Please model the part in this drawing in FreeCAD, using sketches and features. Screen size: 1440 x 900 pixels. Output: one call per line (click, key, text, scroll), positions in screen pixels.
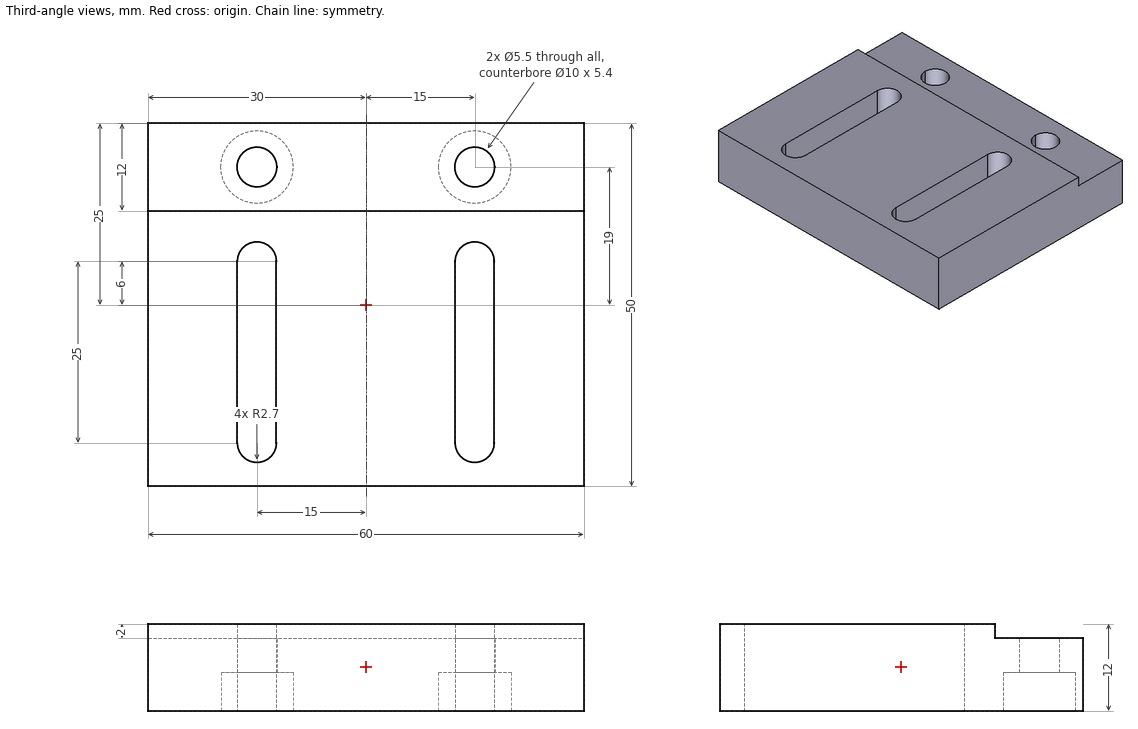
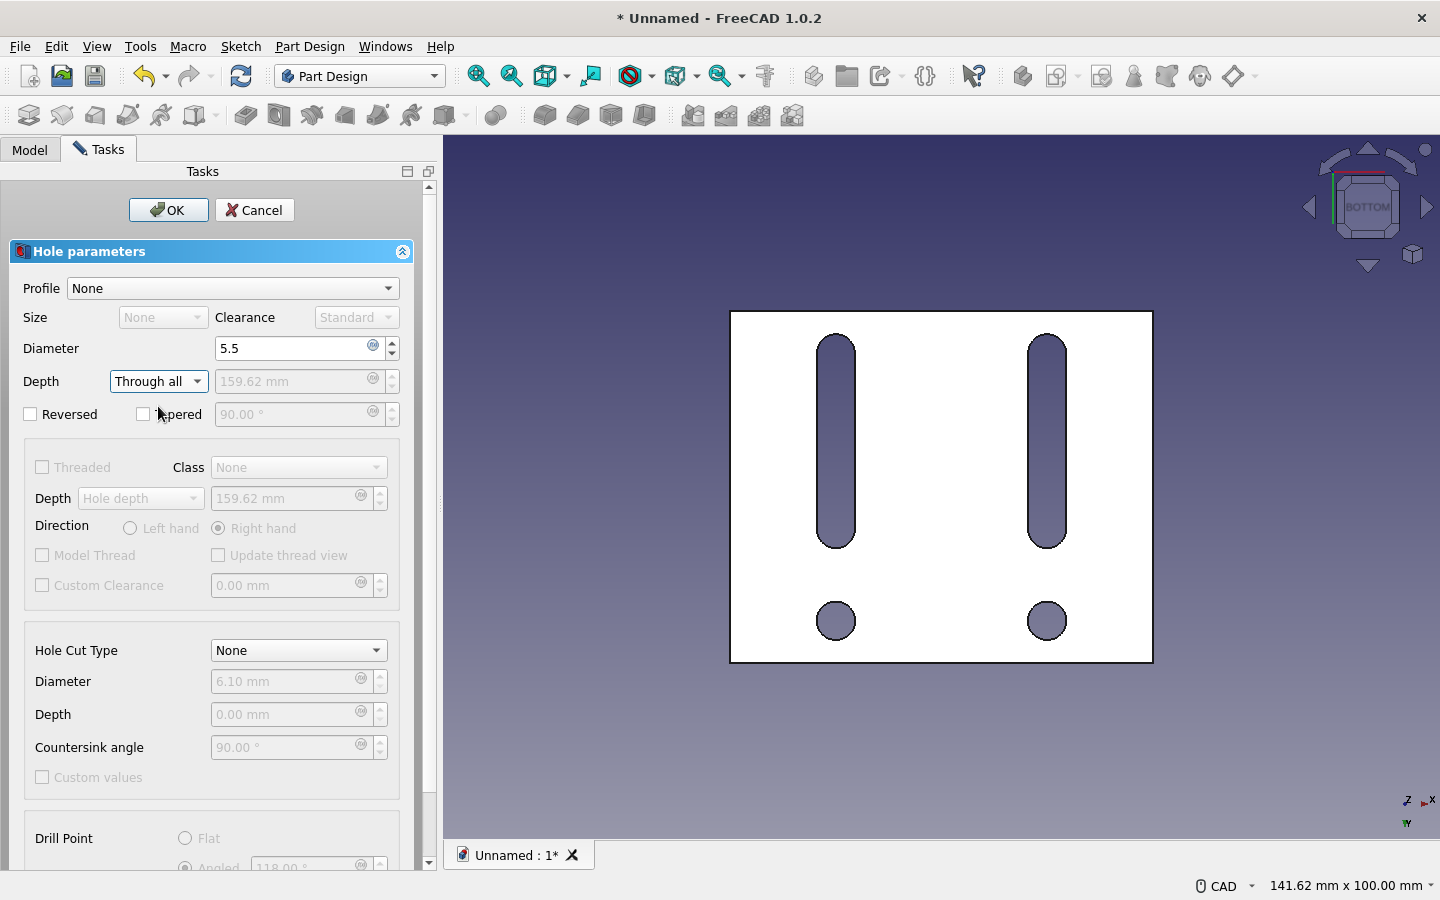
click(300, 650)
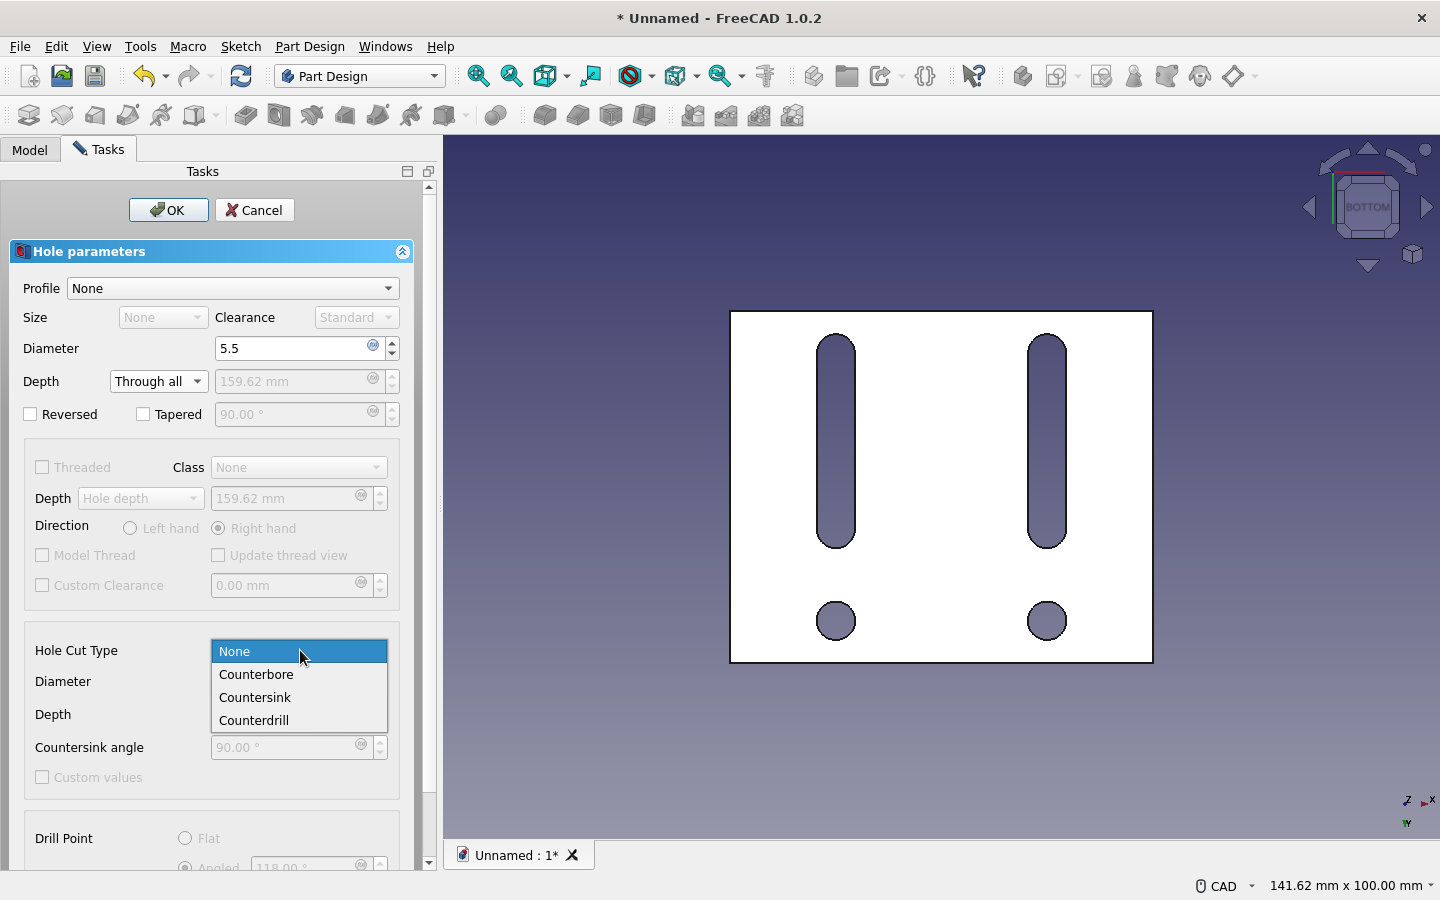
click(298, 674)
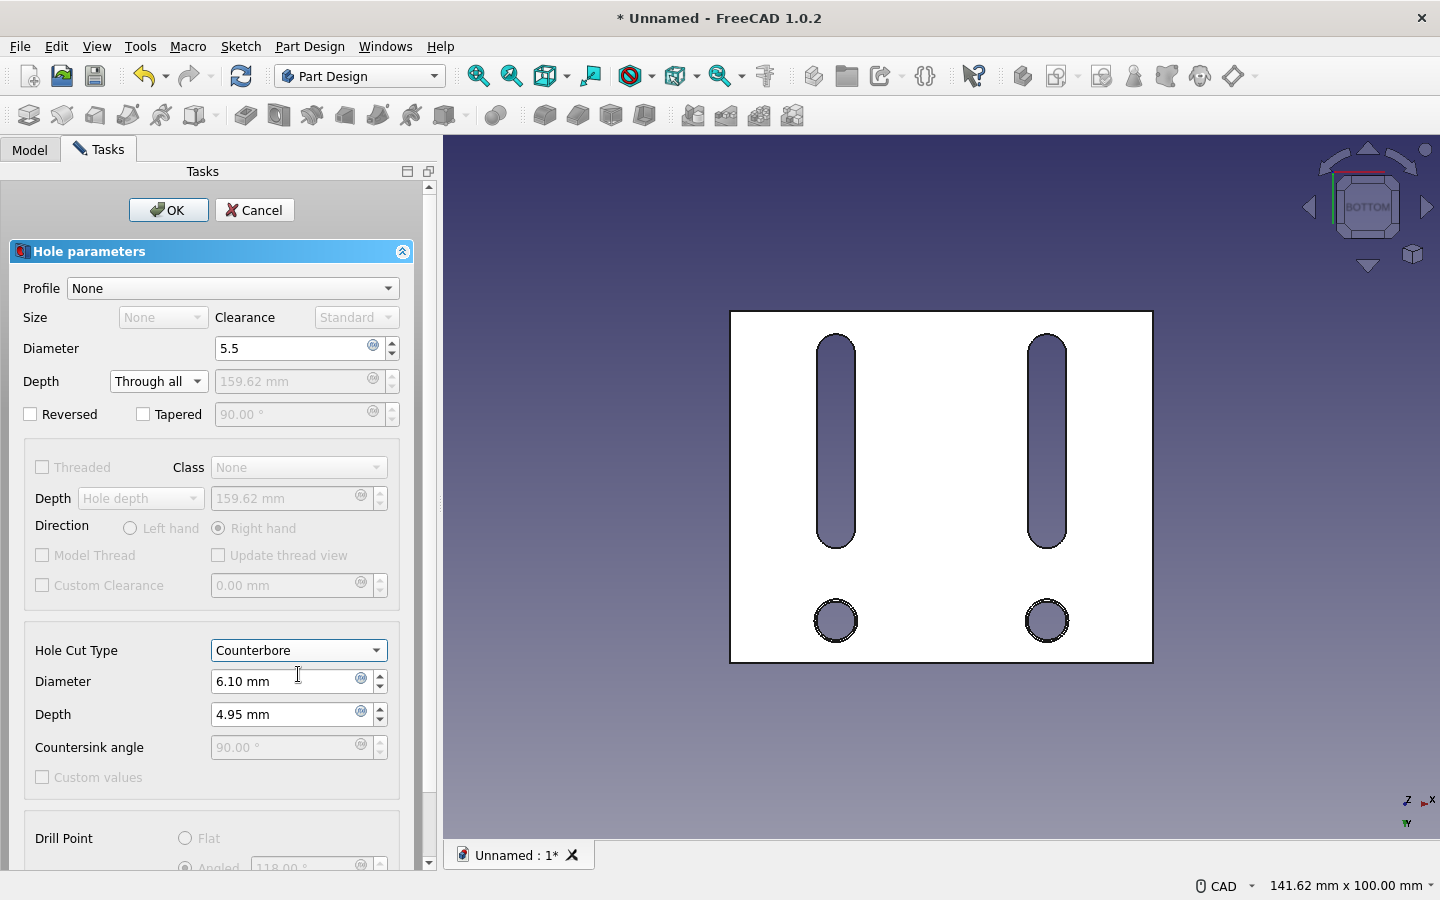
triple_click(292, 682)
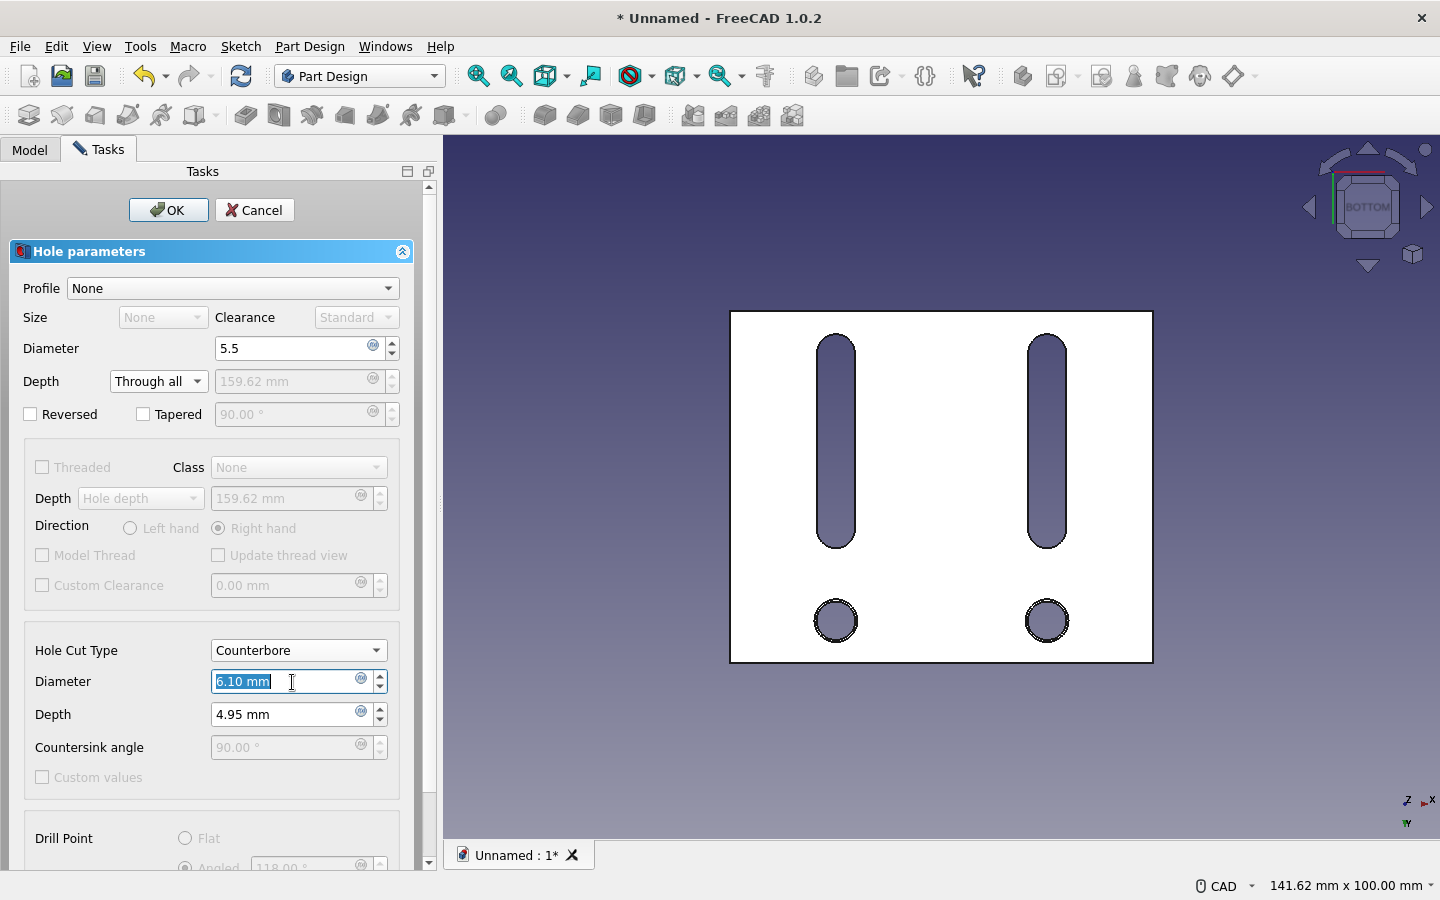
text(10)
key(Tab)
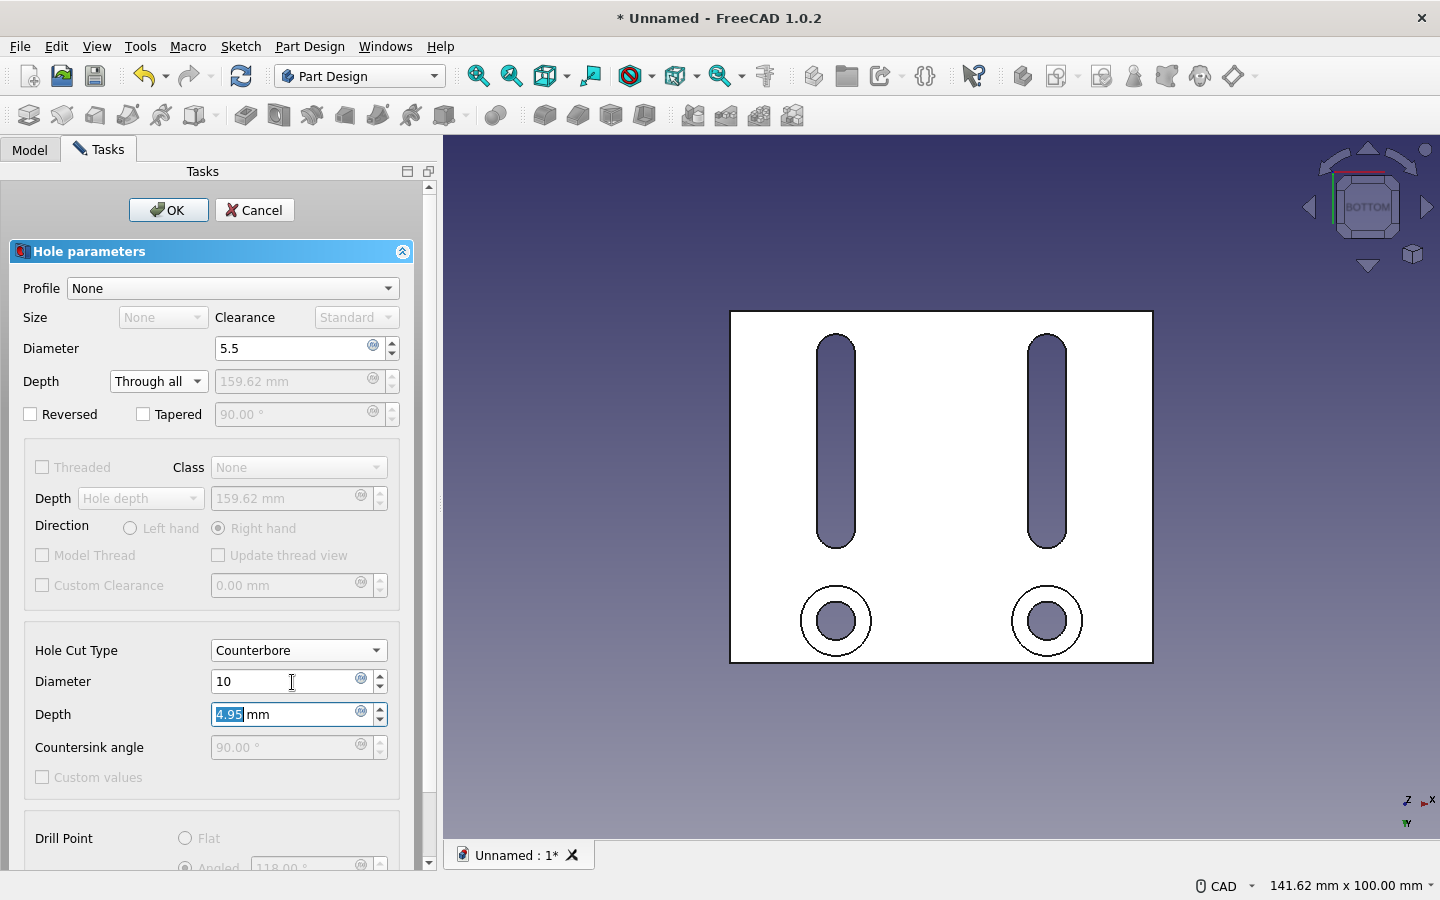
text(5.4)
key(Tab)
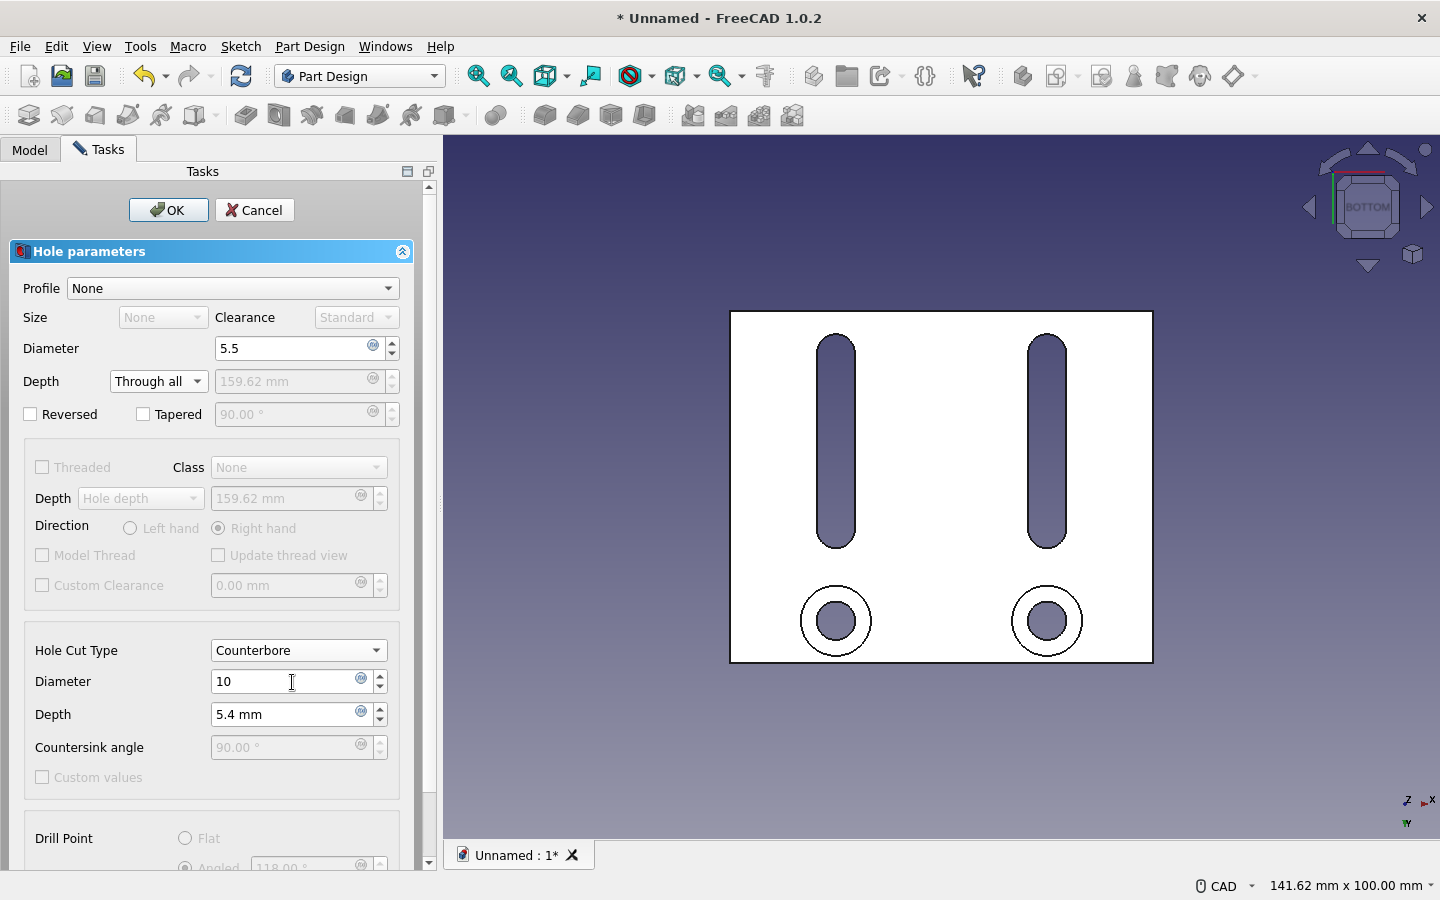
click(169, 210)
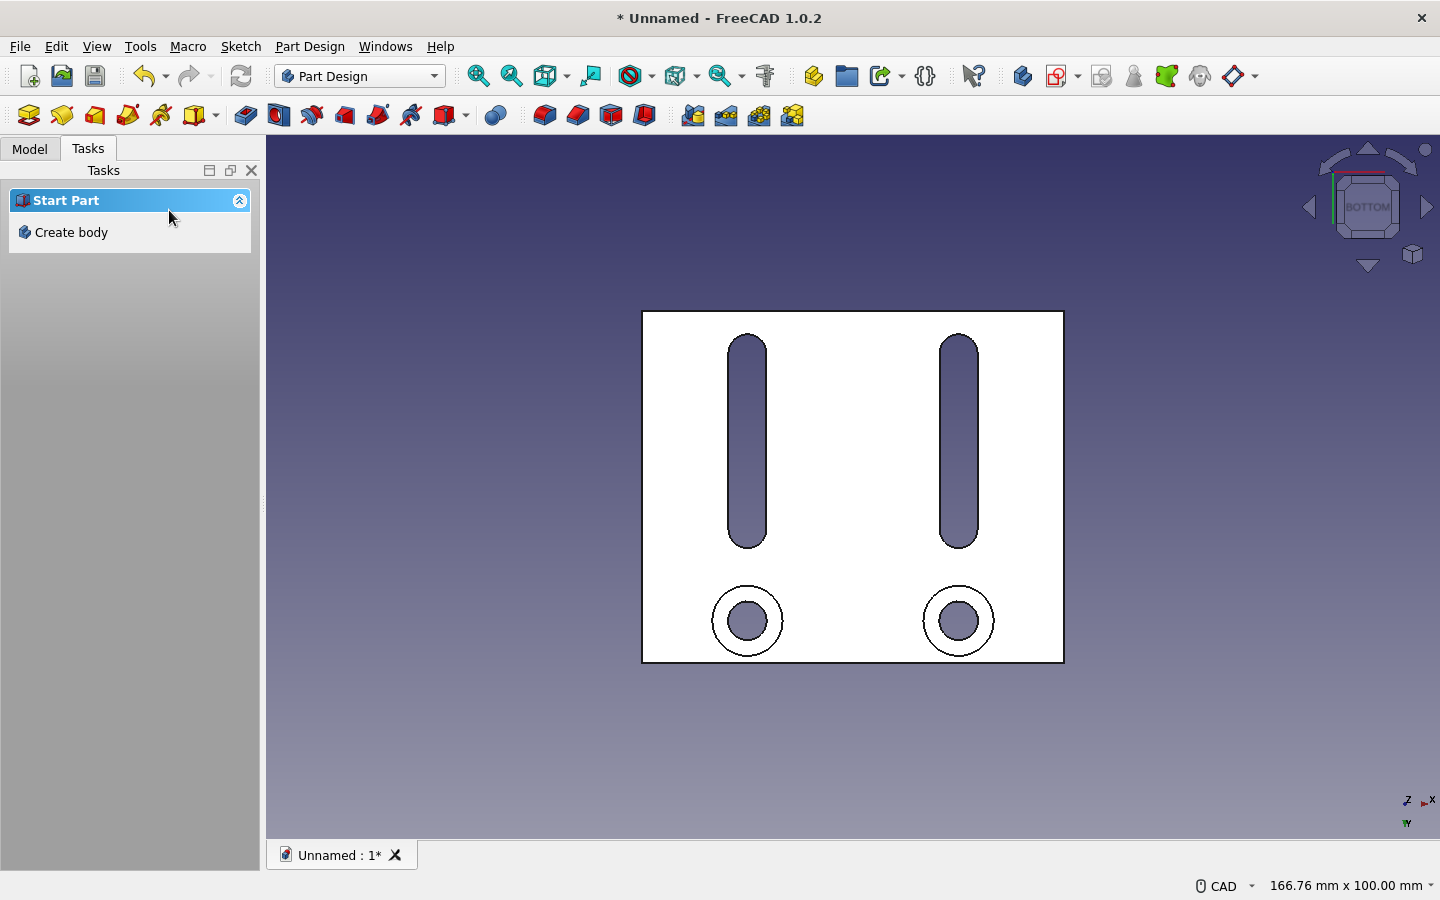
key(0)